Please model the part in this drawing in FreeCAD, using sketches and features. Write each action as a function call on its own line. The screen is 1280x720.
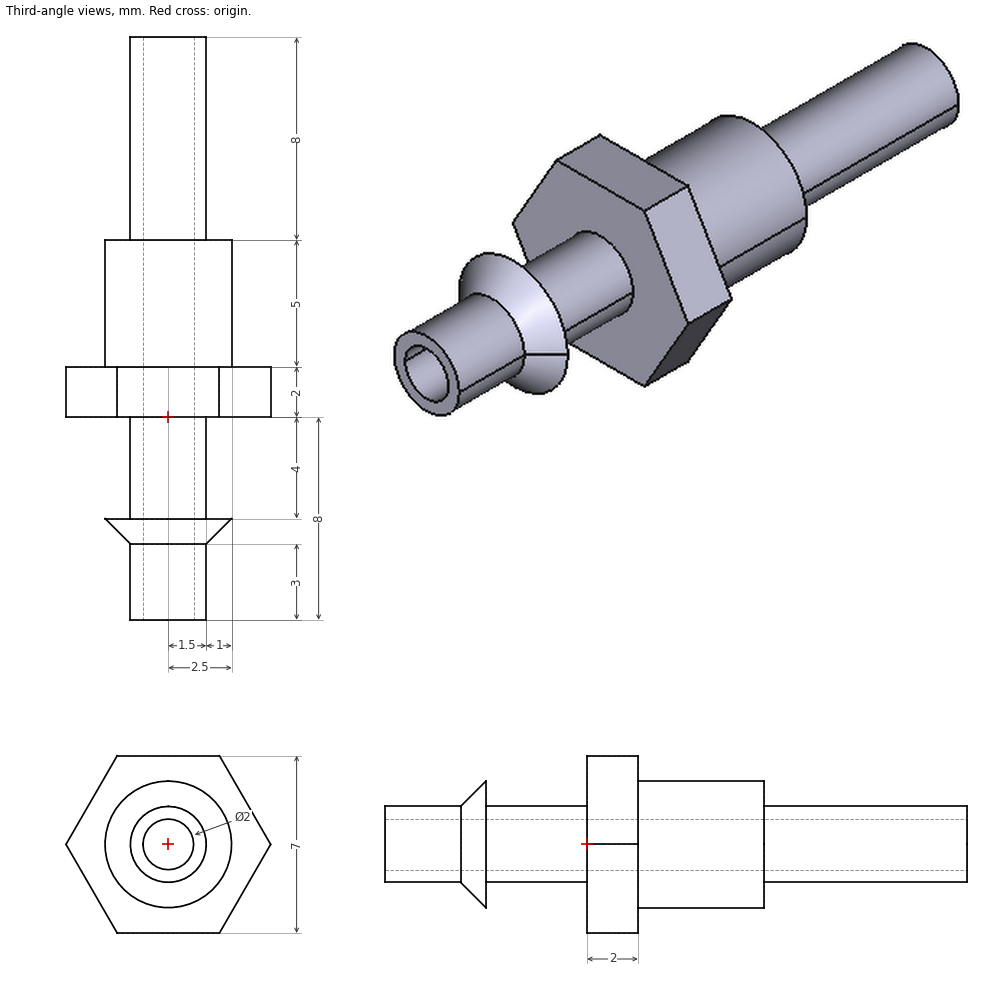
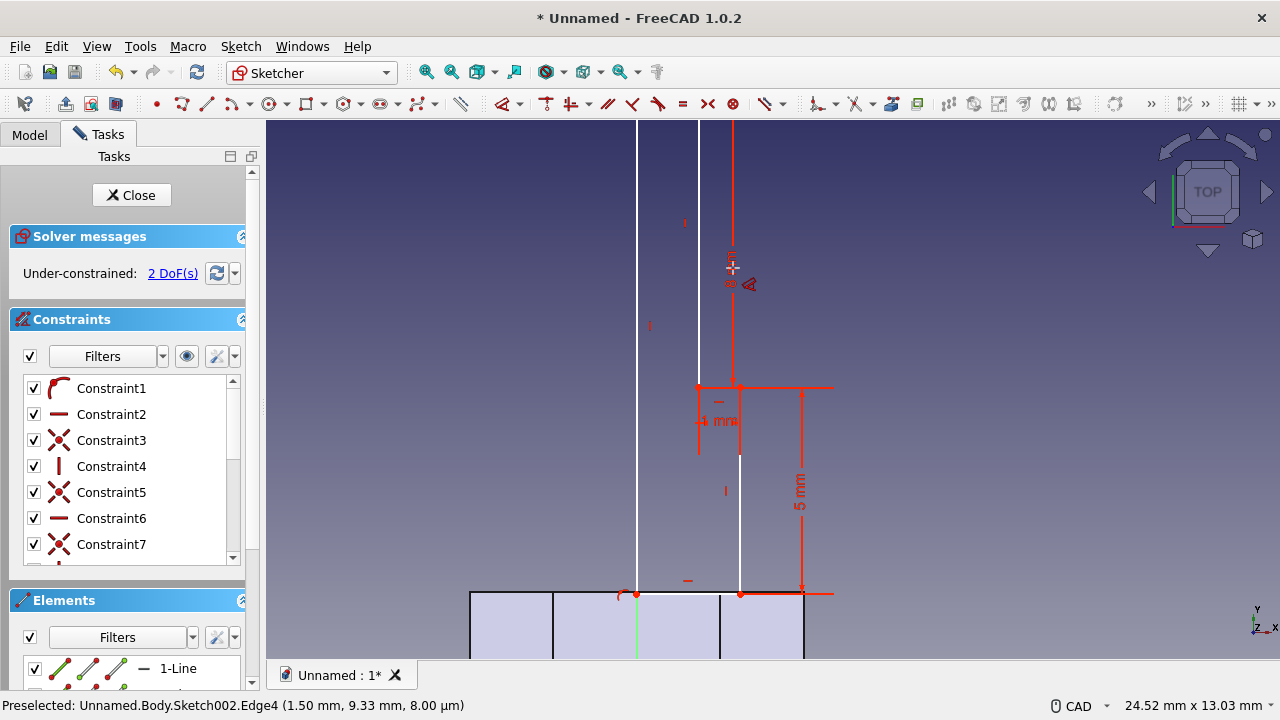
click(637, 594)
click(603, 613)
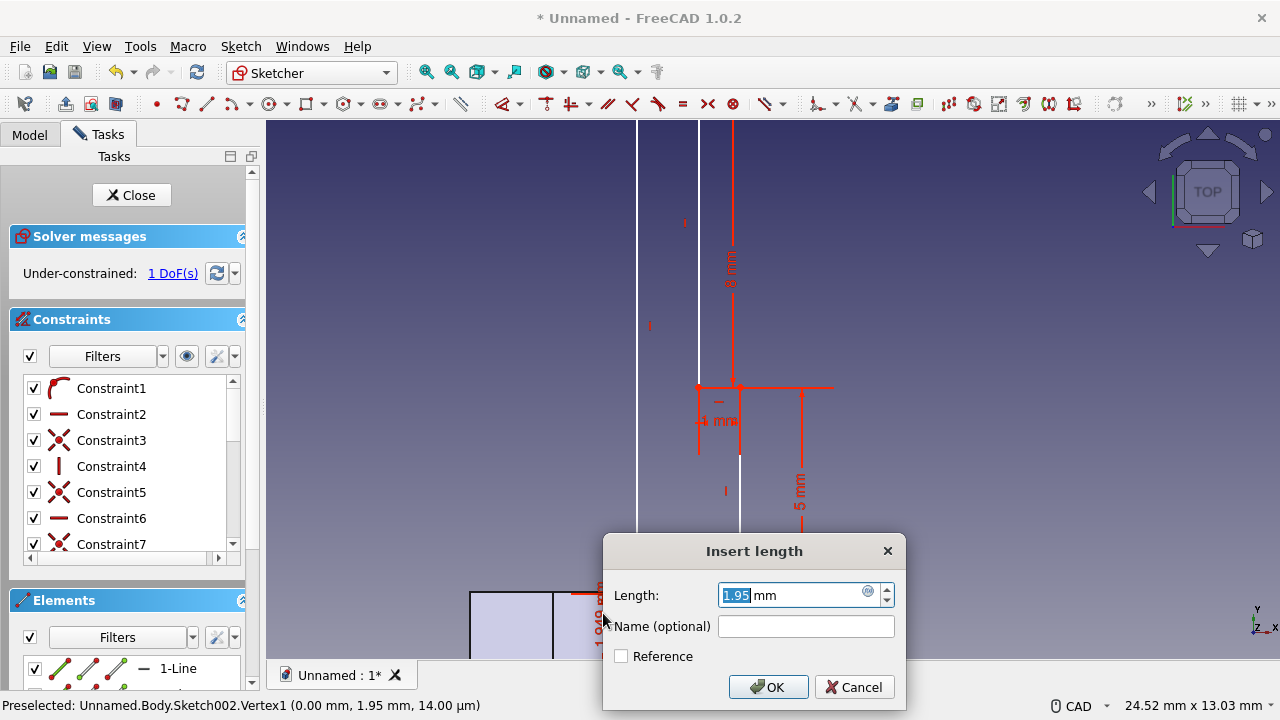
text(2)
key(Return)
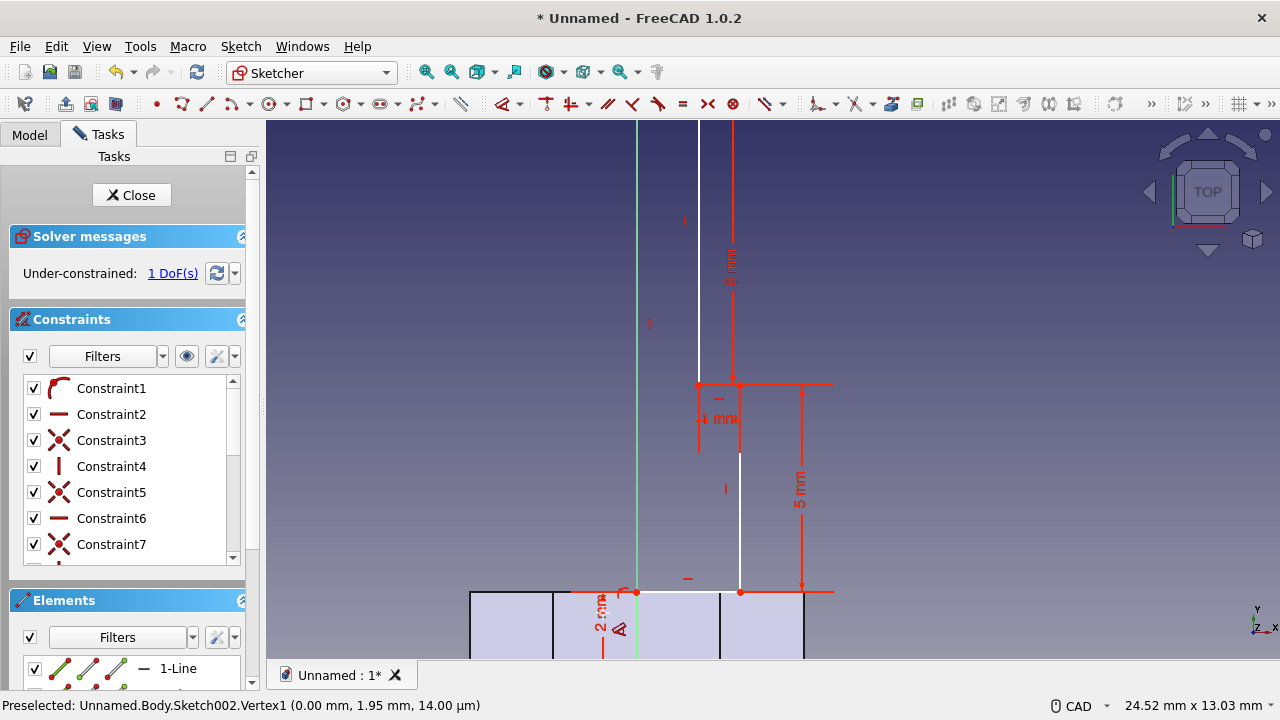
click(668, 592)
click(688, 626)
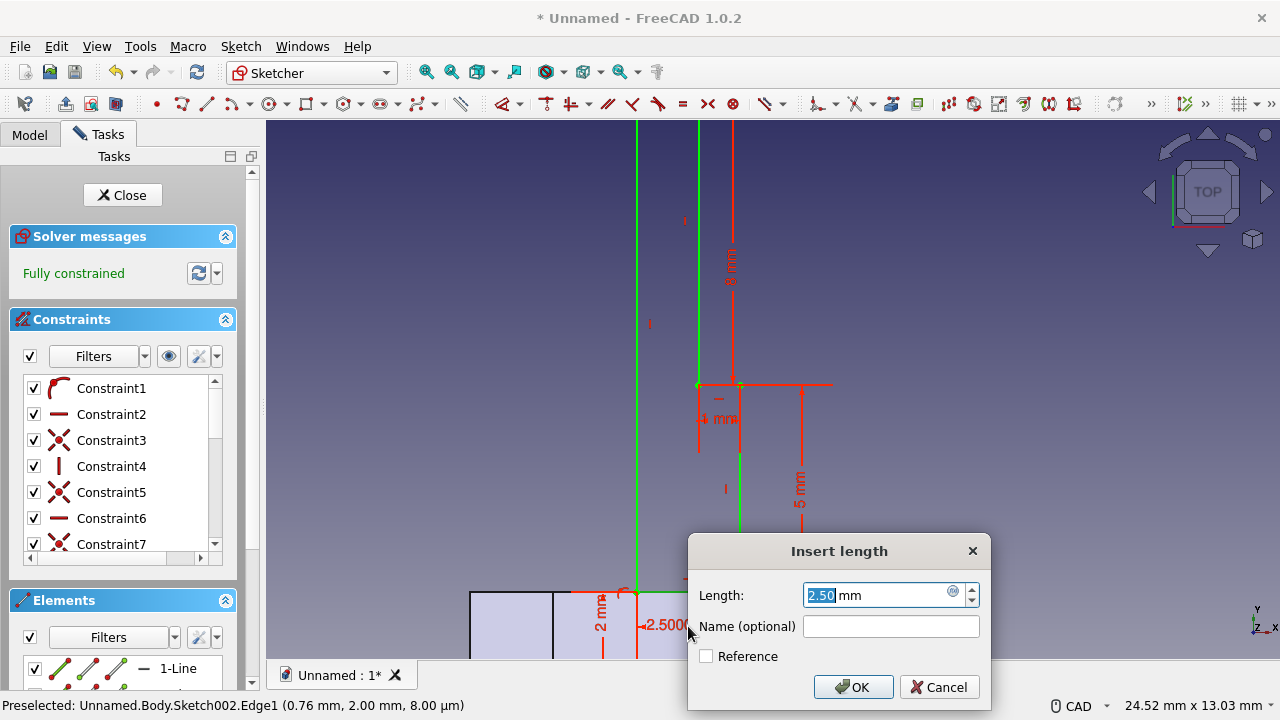
text(2.5)
key(Return)
key(Escape)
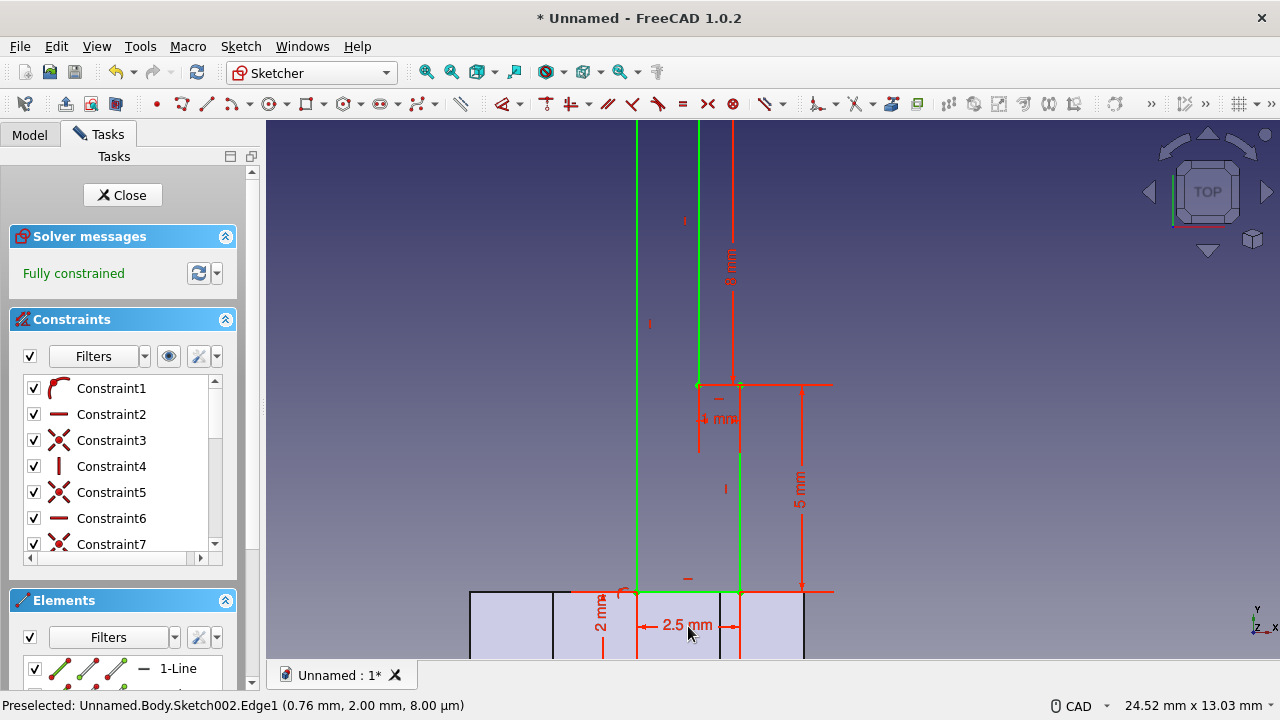
click(123, 195)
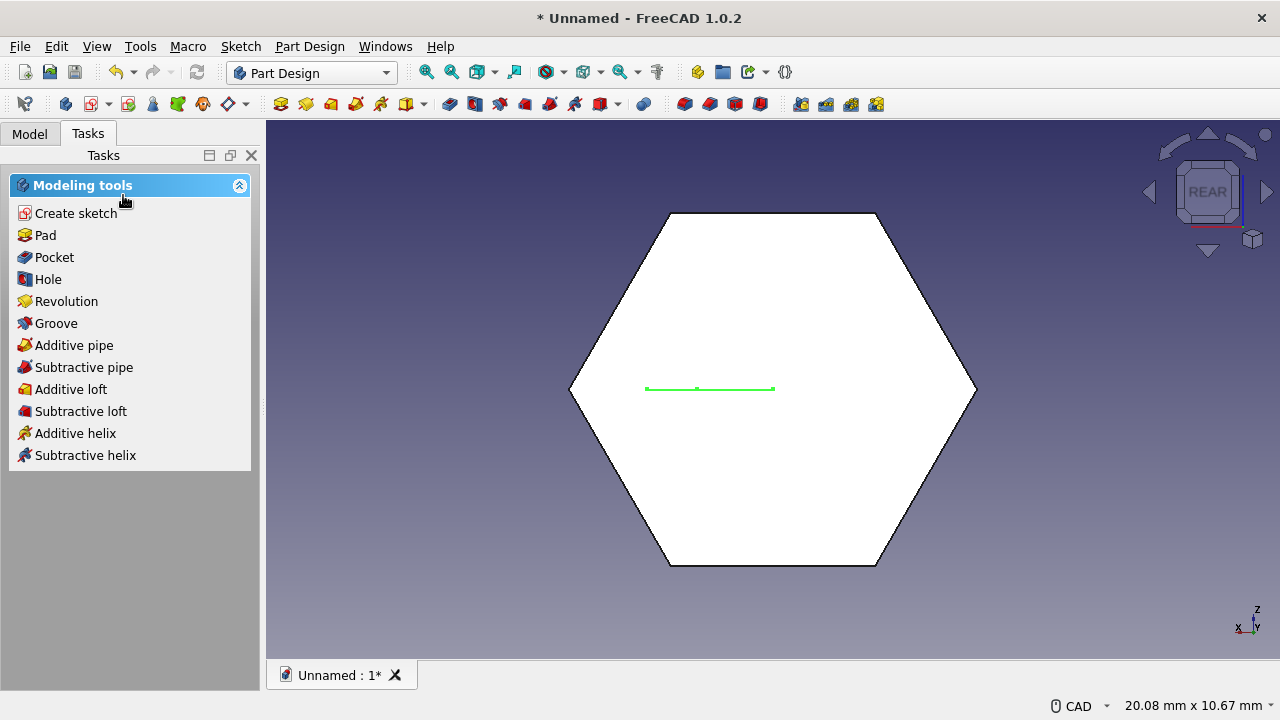
click(306, 104)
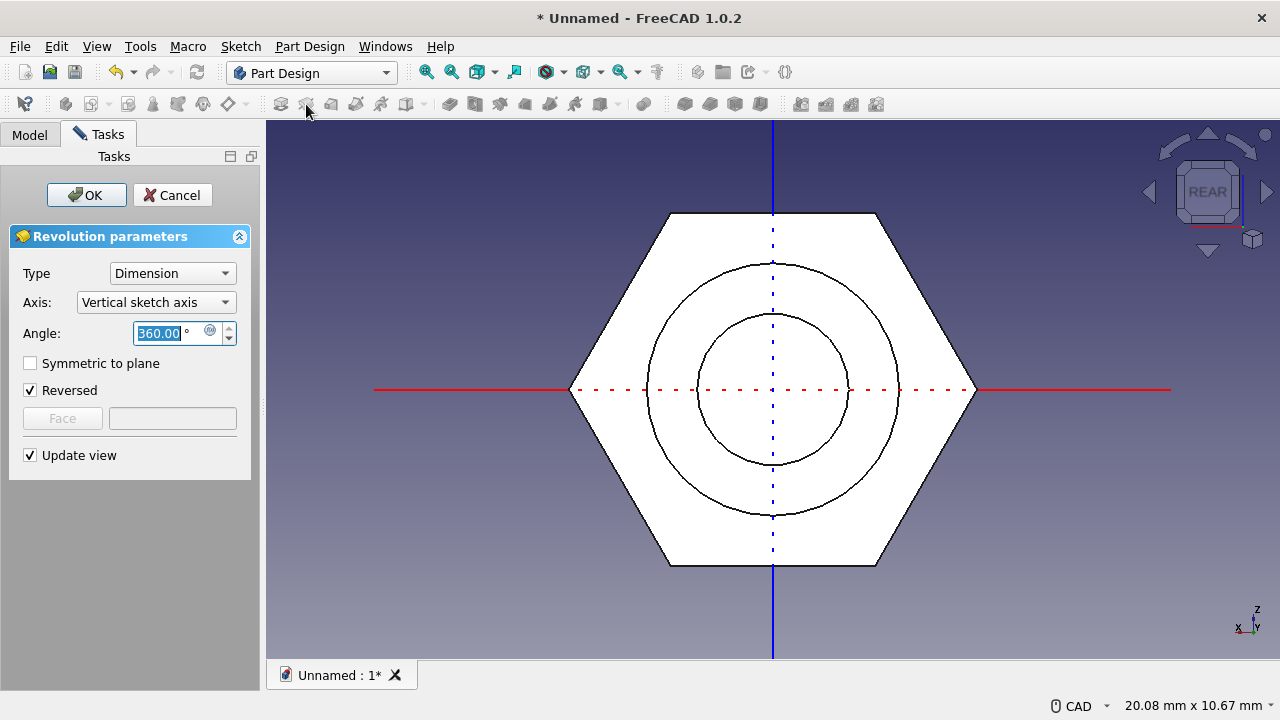
click(87, 195)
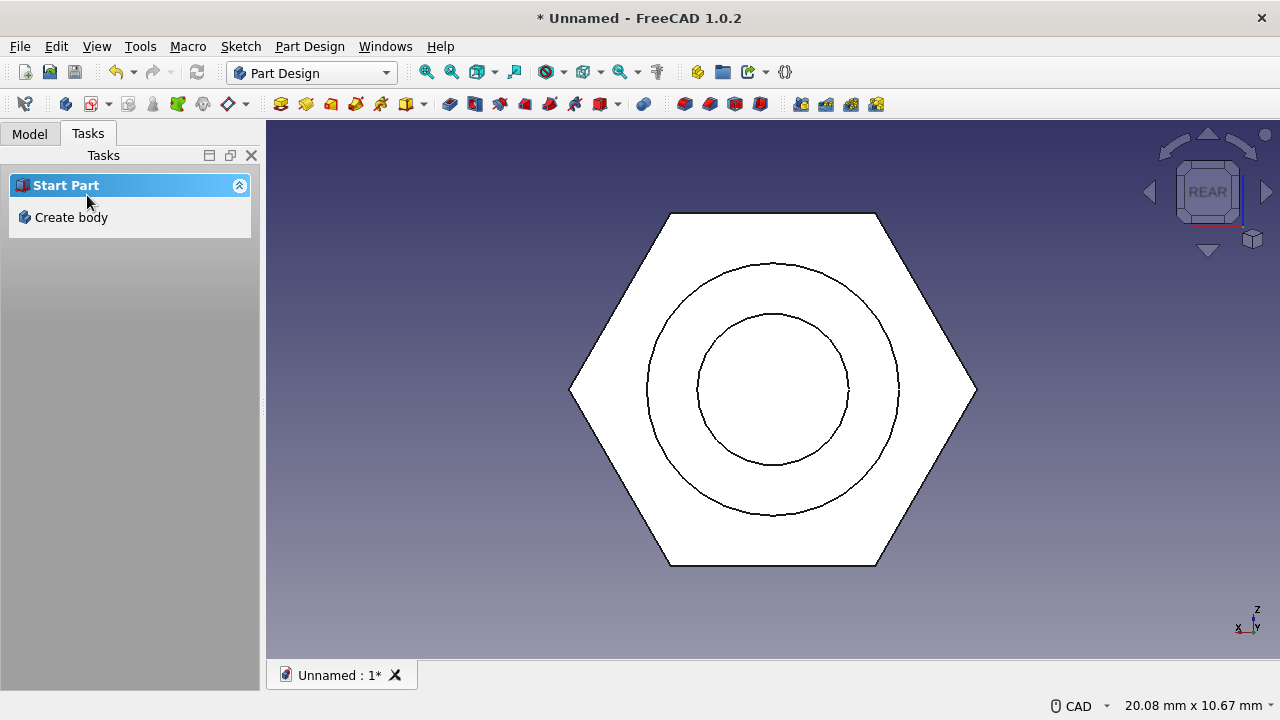
click(773, 388)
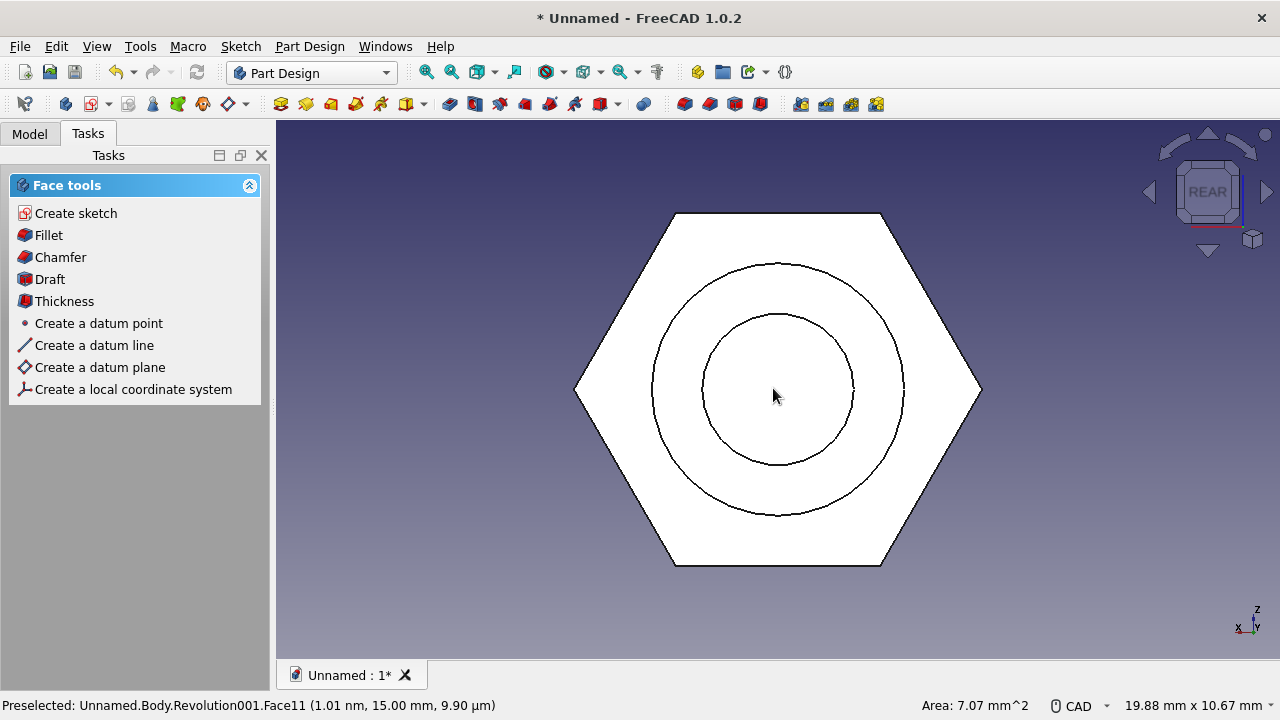
click(90, 104)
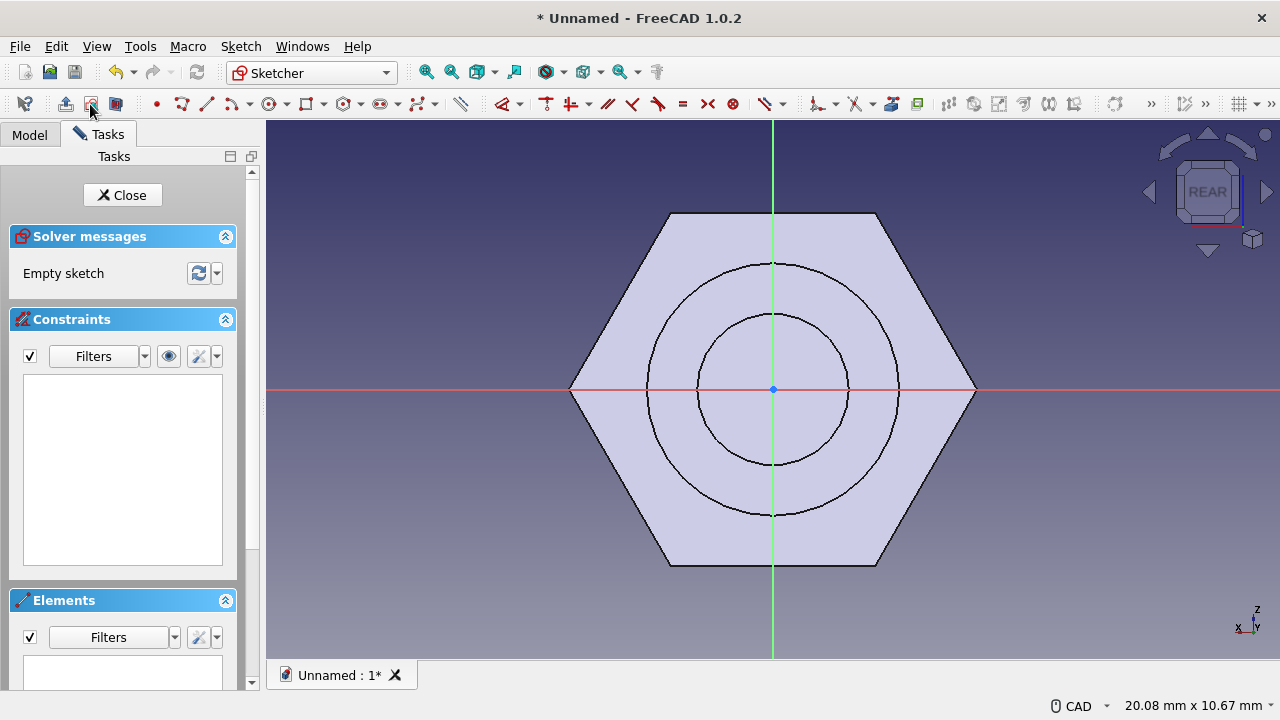
scroll(803, 390, up, 6)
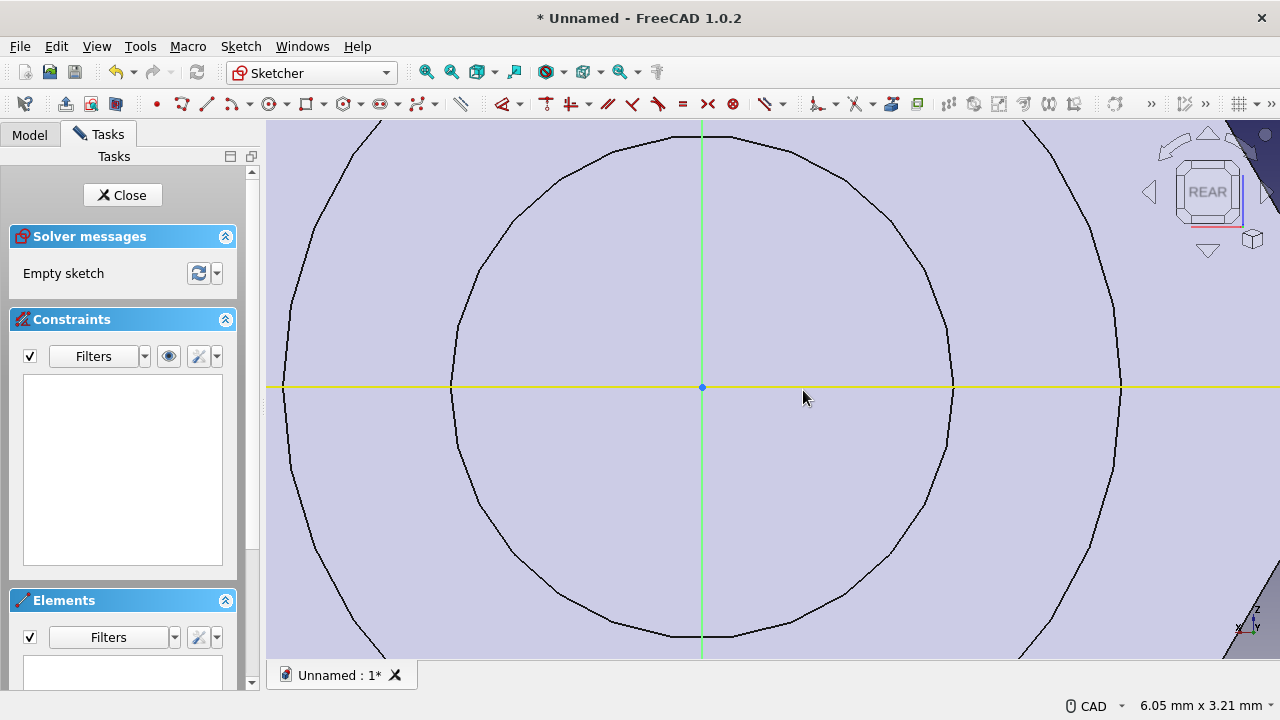
click(268, 104)